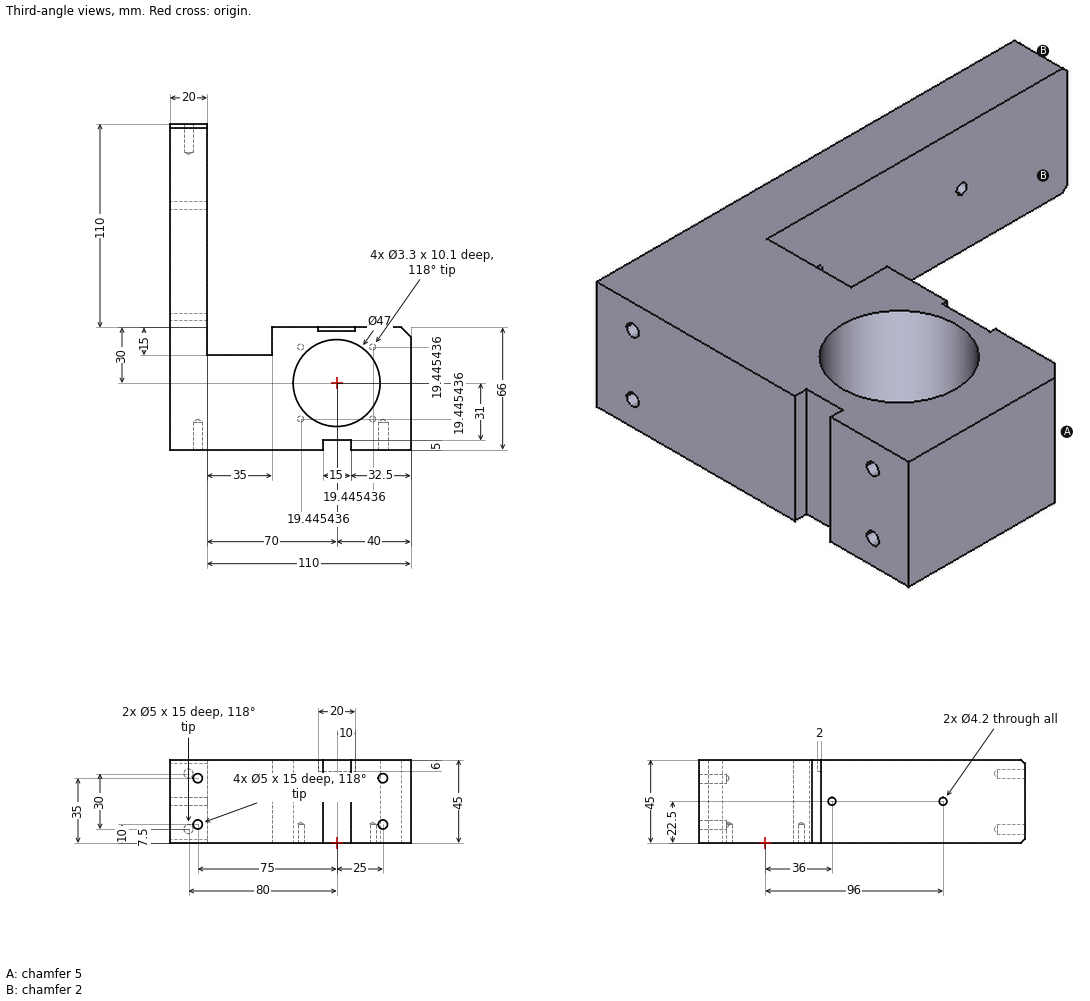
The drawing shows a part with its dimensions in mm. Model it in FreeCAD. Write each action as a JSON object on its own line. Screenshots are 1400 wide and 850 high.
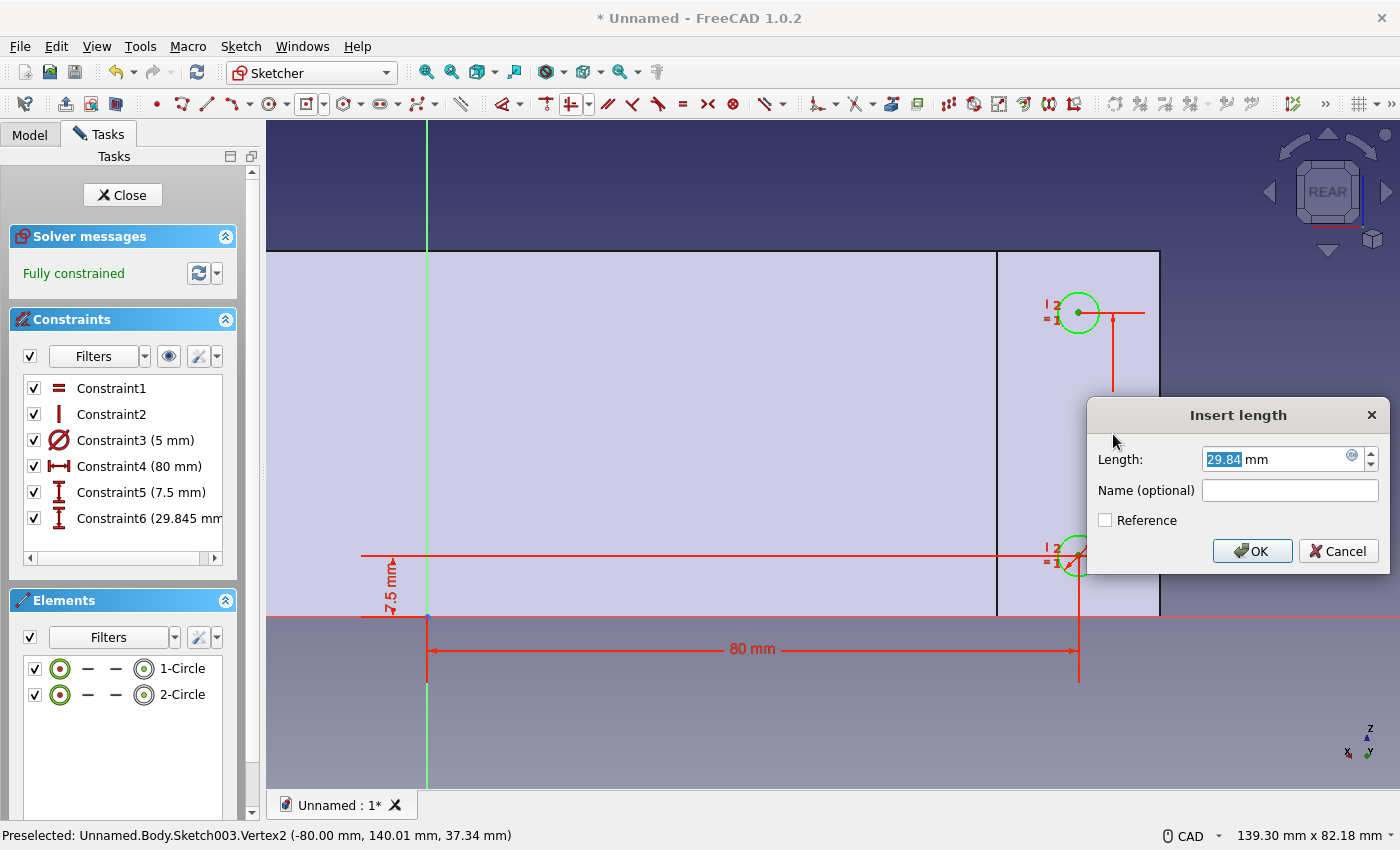
{"action": "type", "text": "30"}
{"action": "key", "text": "Return"}
{"action": "key", "text": "Escape"}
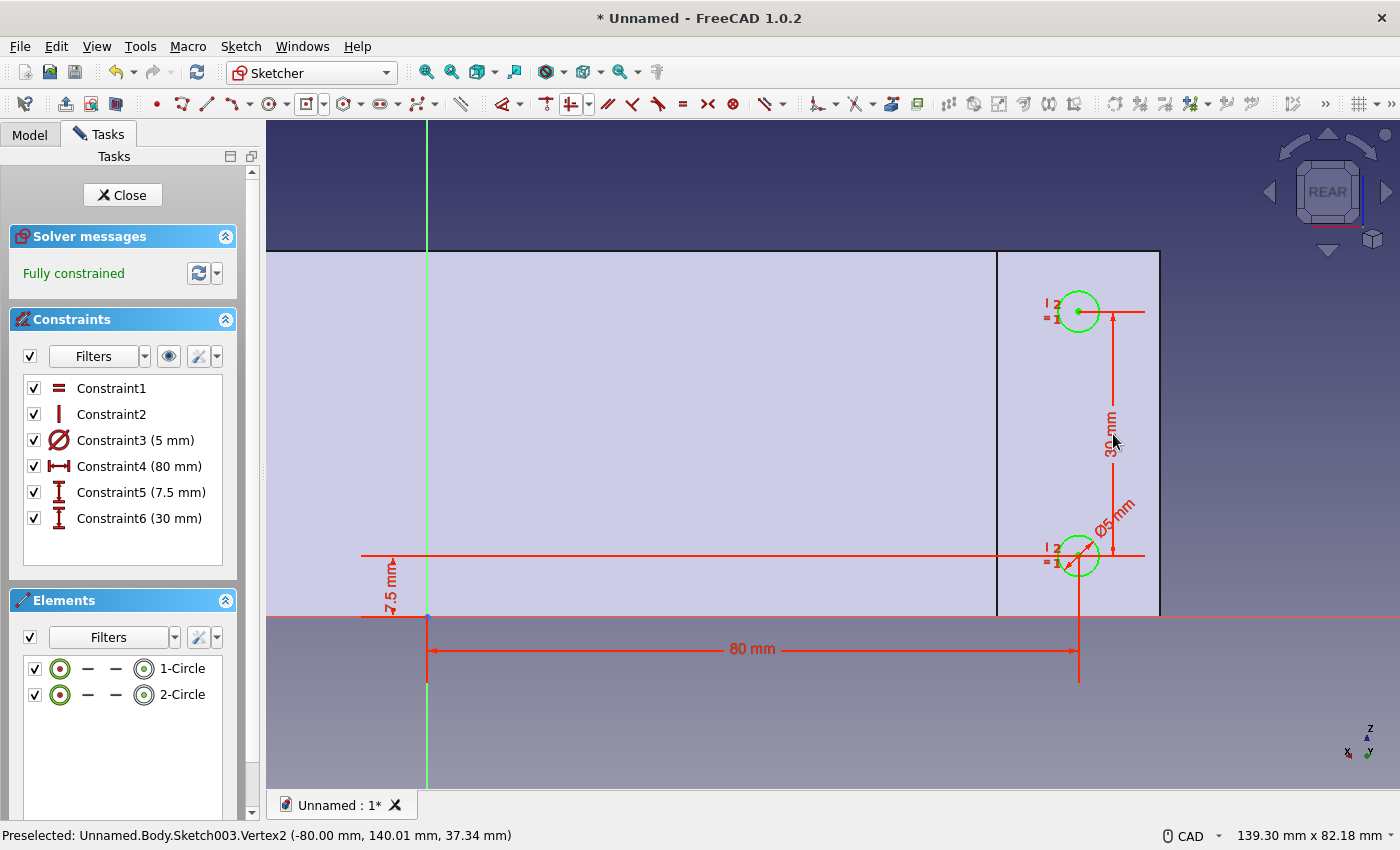
{"action": "left_click", "coordinate": [123, 195]}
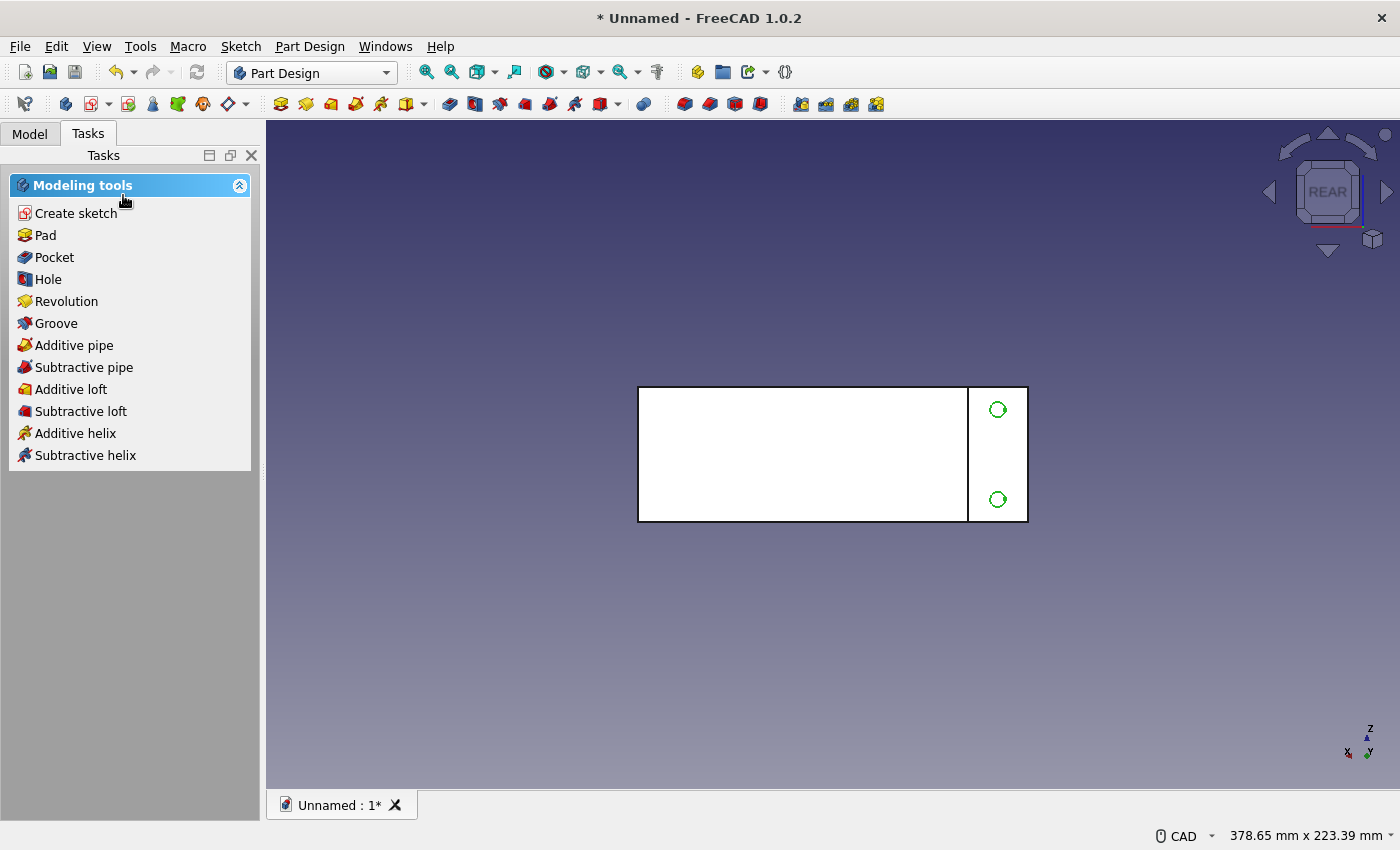
{"action": "left_click", "coordinate": [475, 104]}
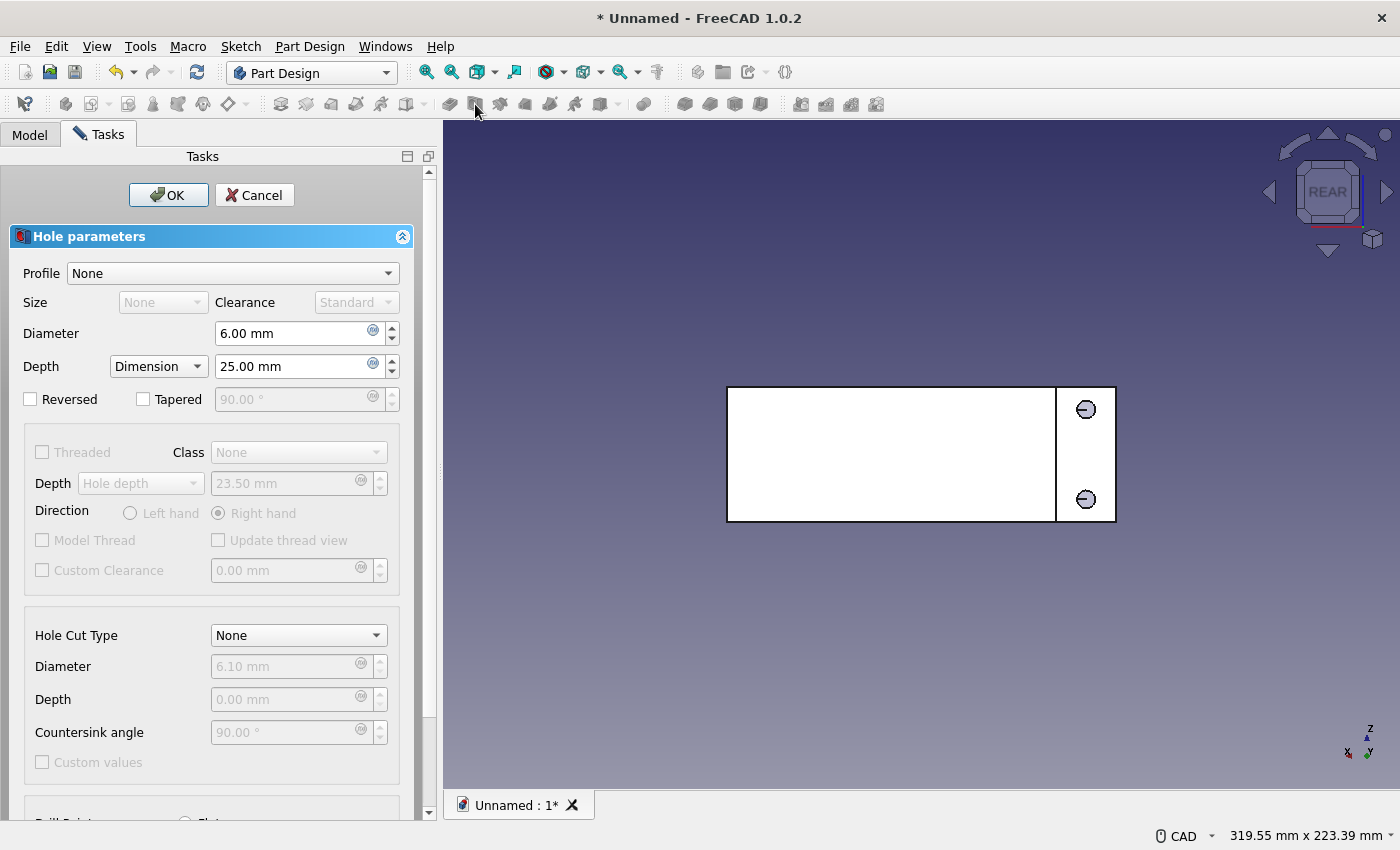
{"action": "triple_click", "coordinate": [300, 334]}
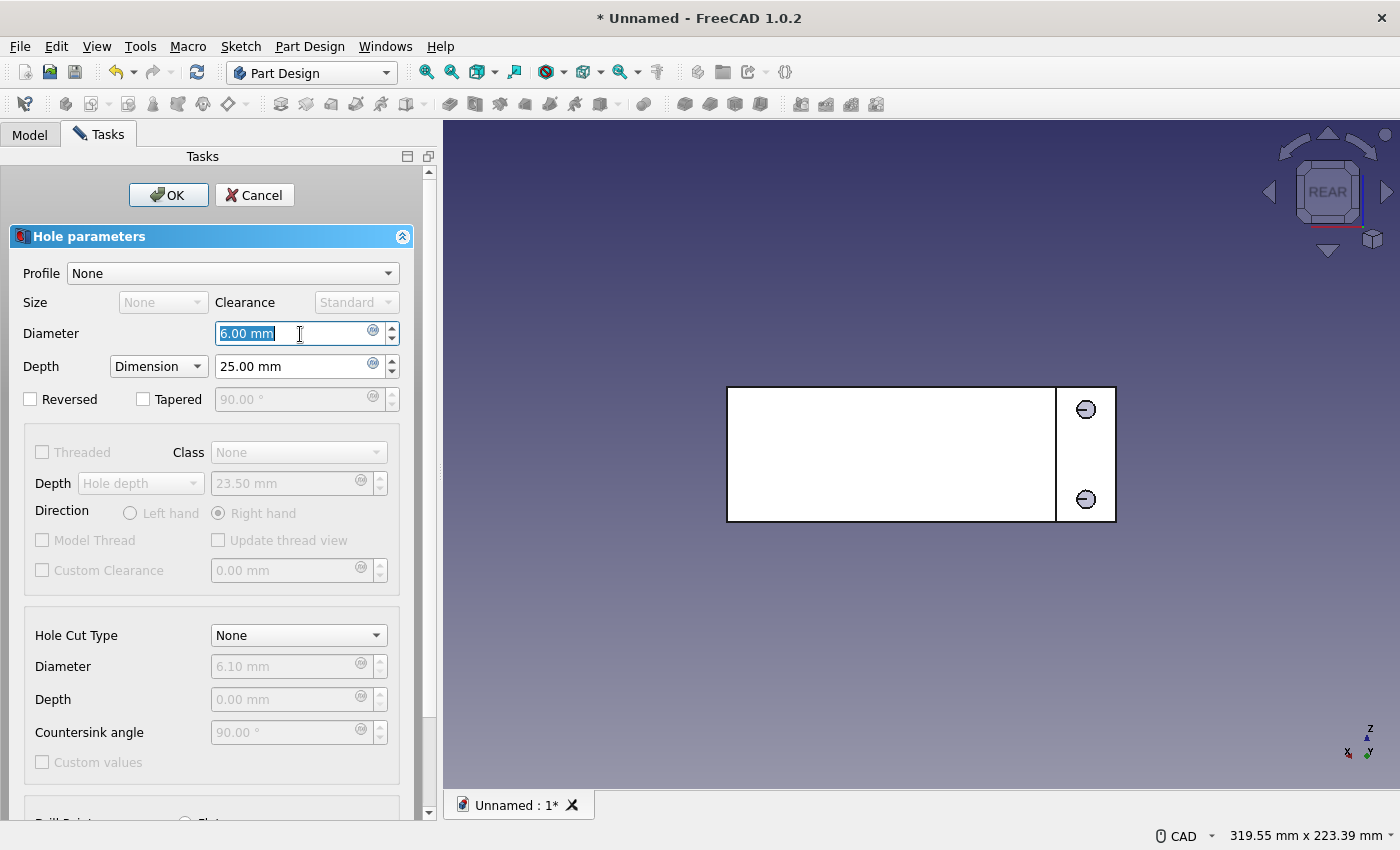
{"action": "type", "text": "5"}
{"action": "key", "text": "Tab"}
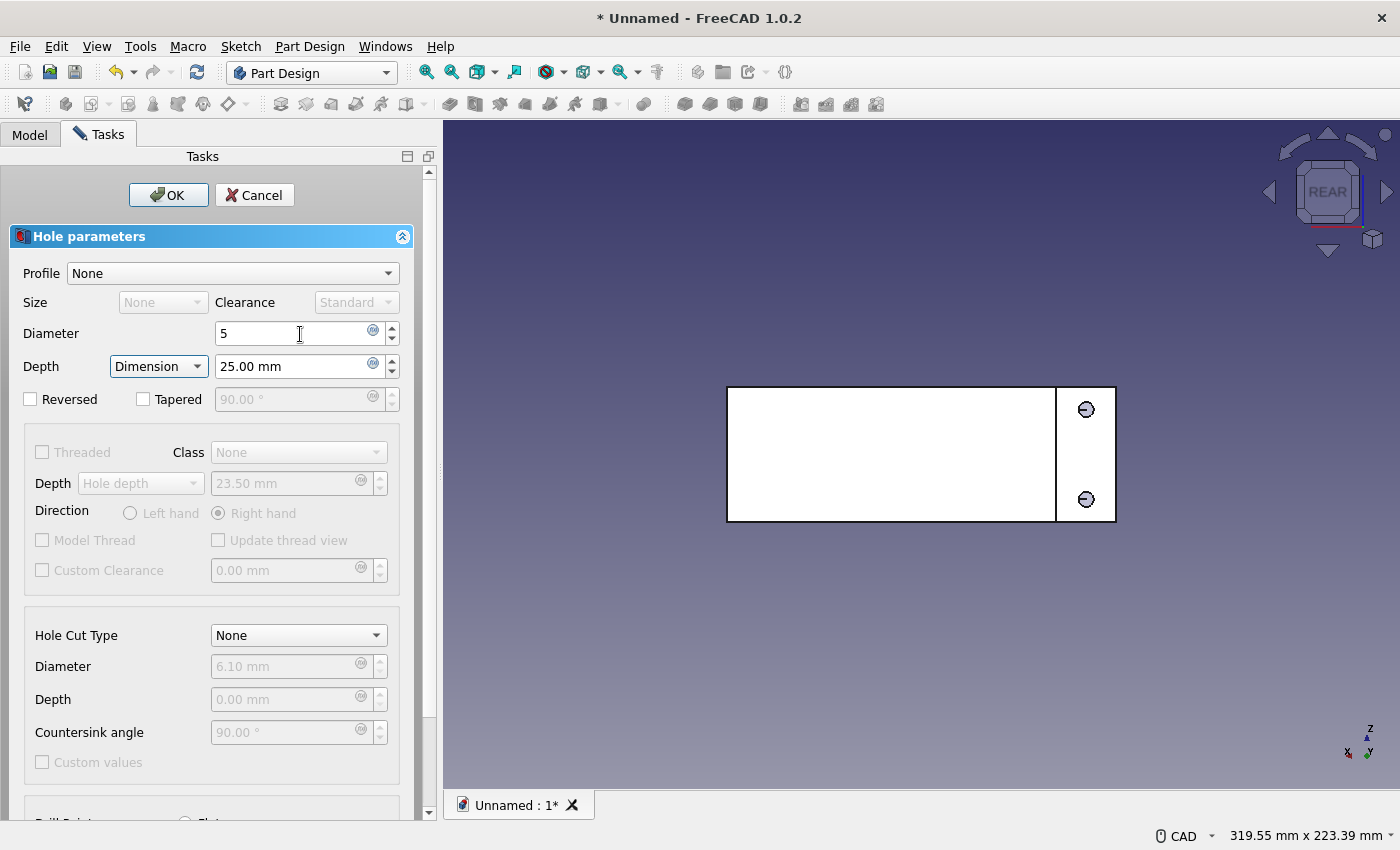
{"action": "triple_click", "coordinate": [300, 366]}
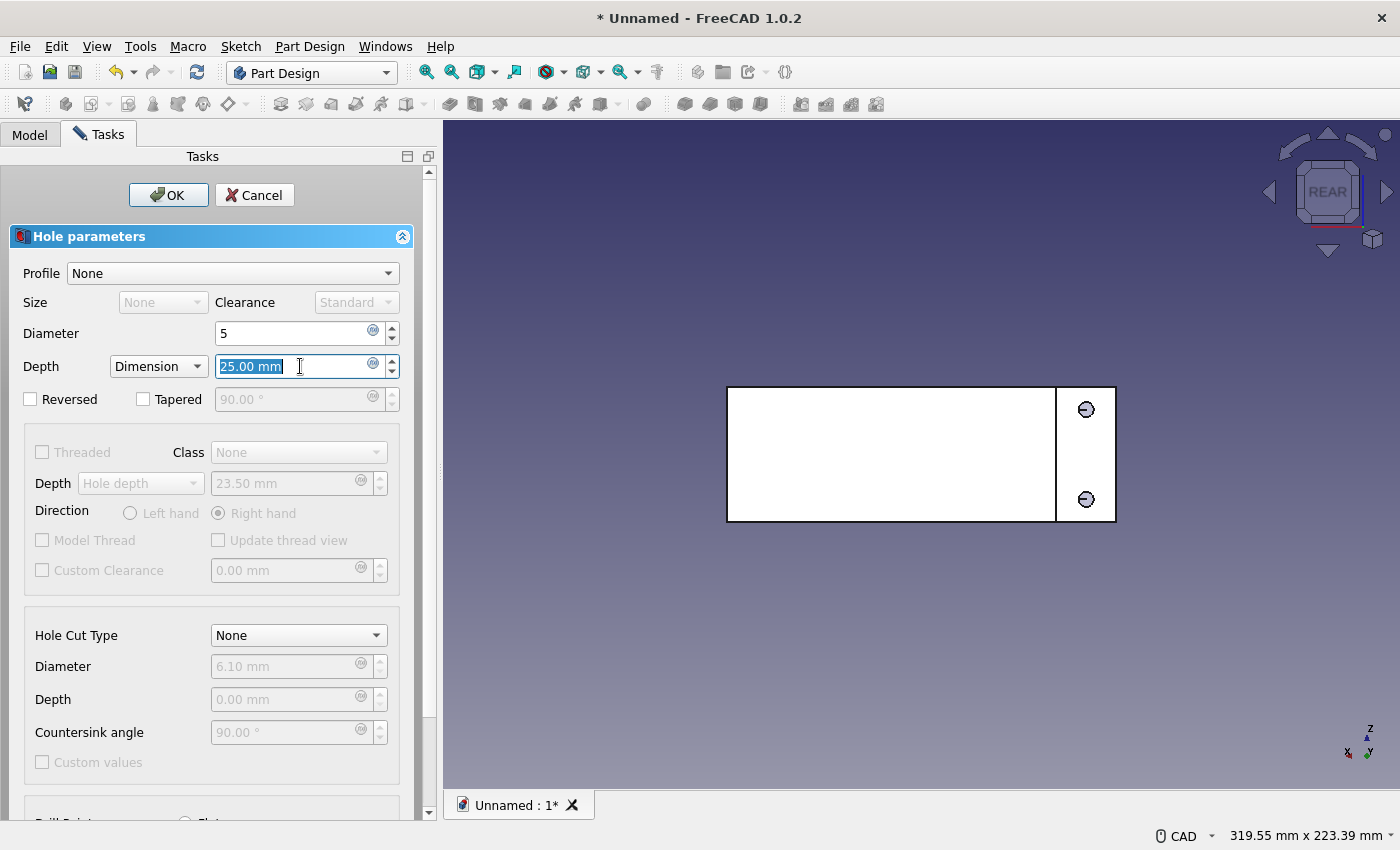
{"action": "type", "text": "15"}
{"action": "key", "text": "Tab"}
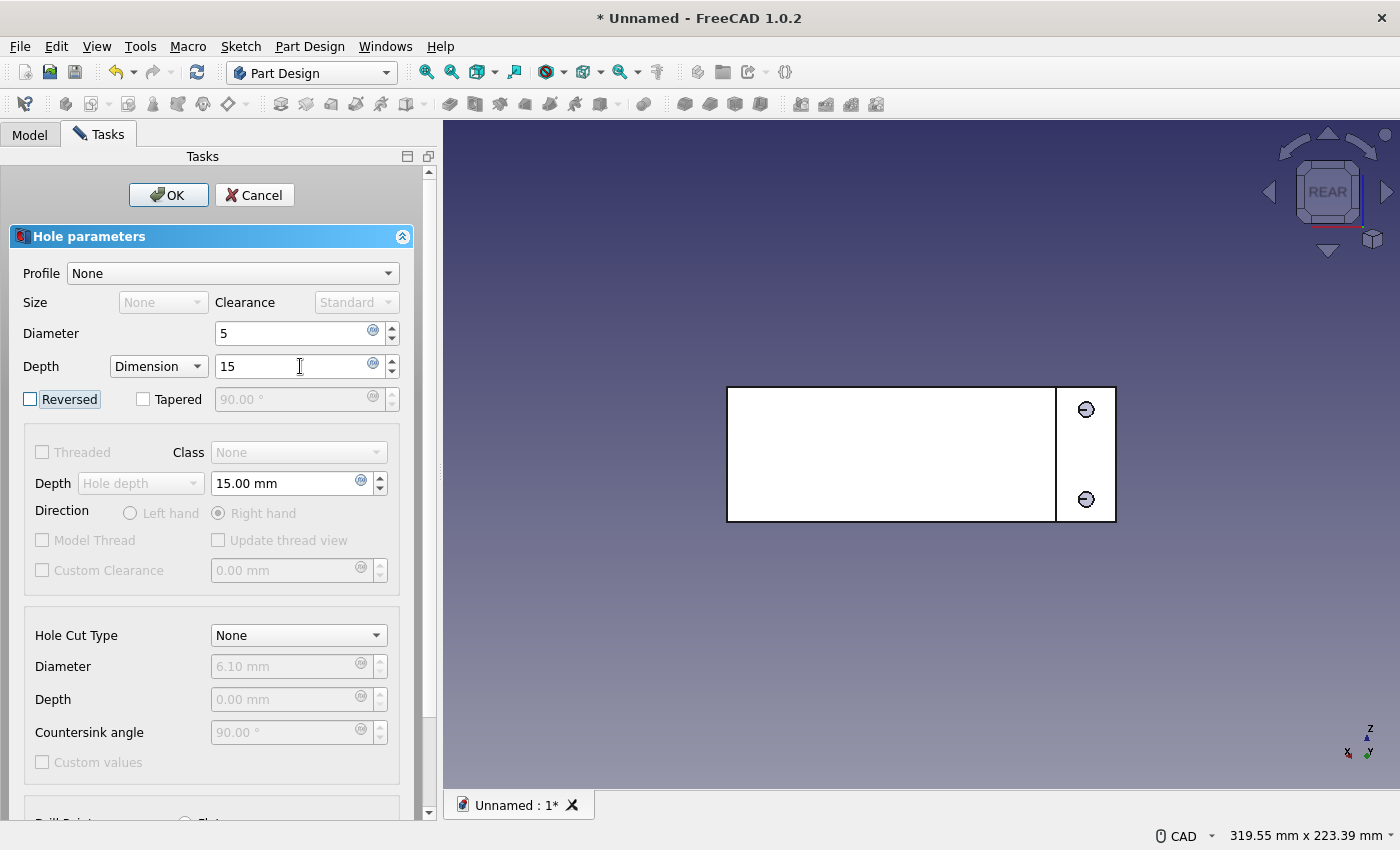
{"action": "left_click", "coordinate": [169, 195]}